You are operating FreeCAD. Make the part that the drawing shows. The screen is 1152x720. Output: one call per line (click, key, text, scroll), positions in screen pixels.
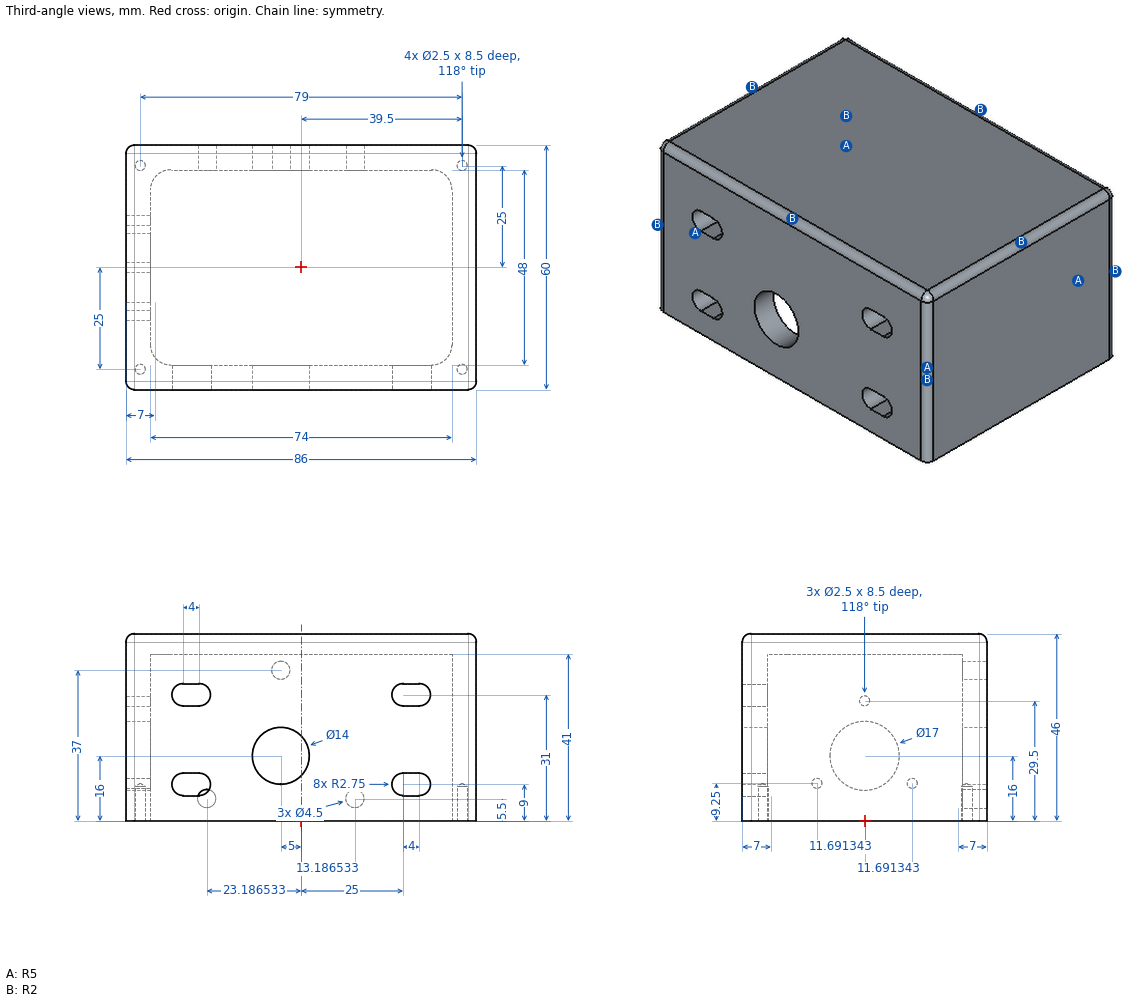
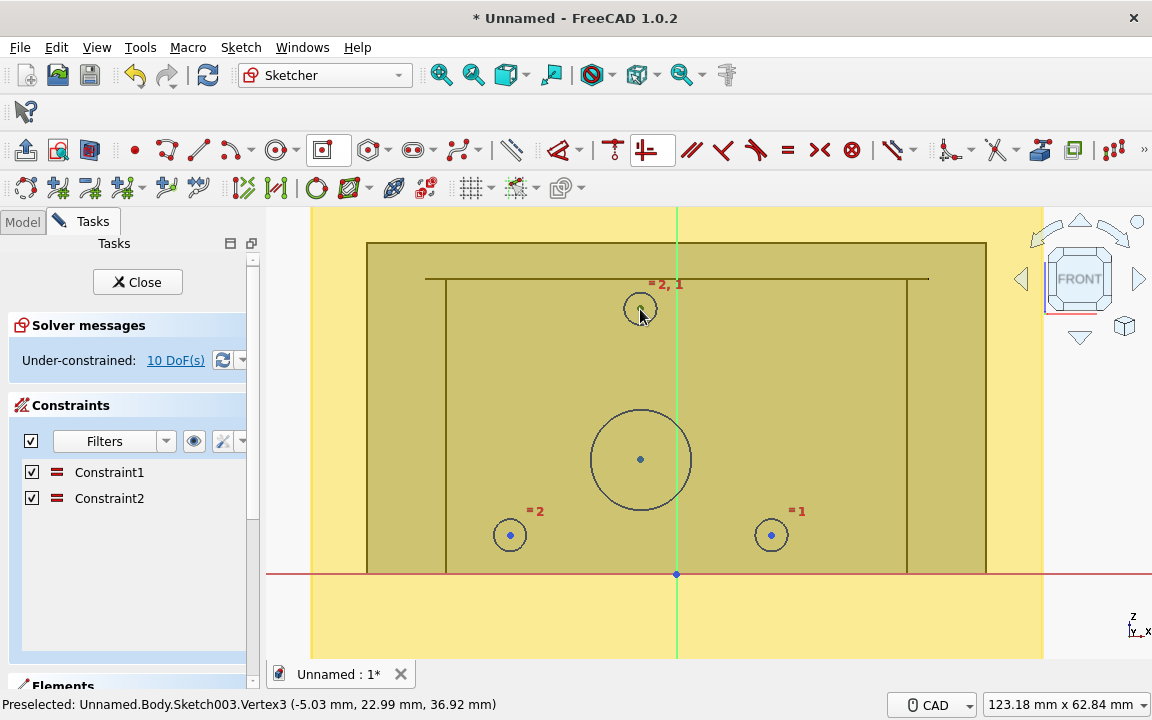
key(v)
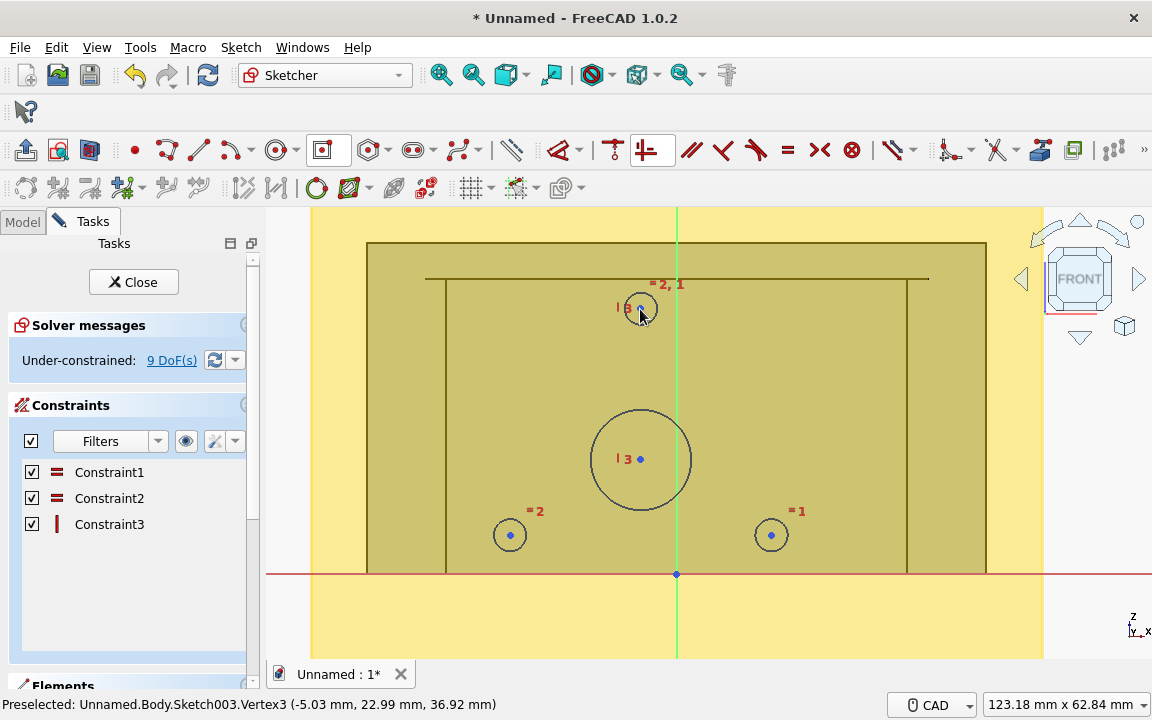
click(772, 535)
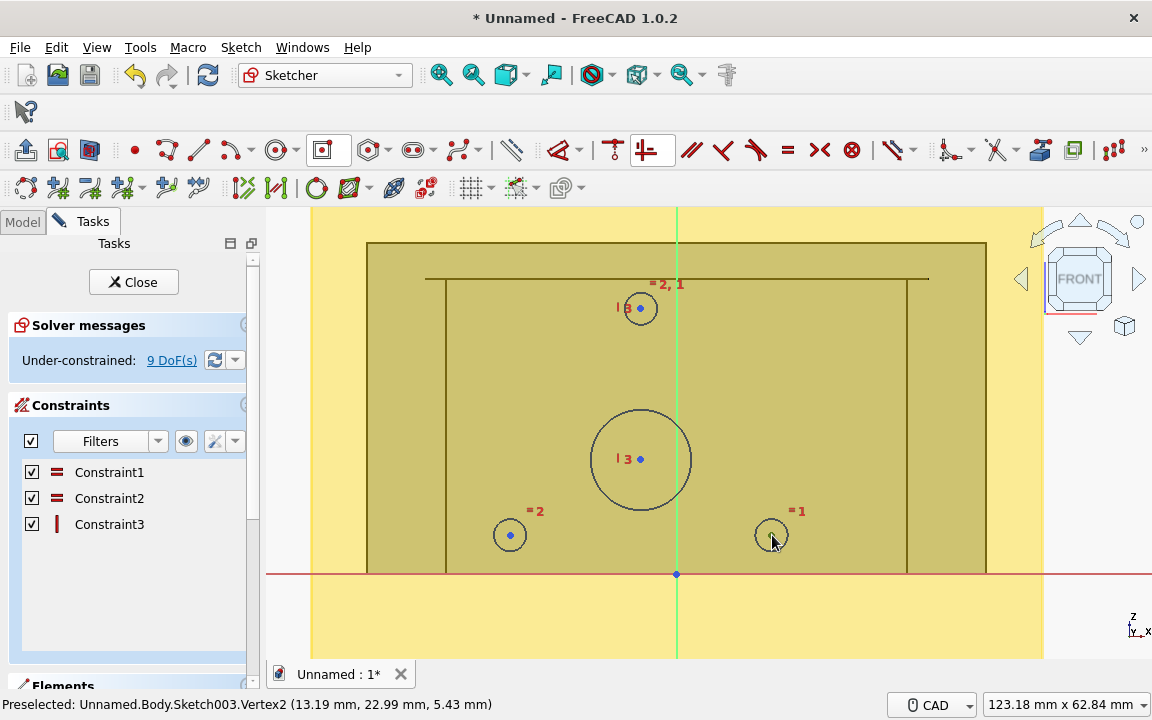
click(510, 535)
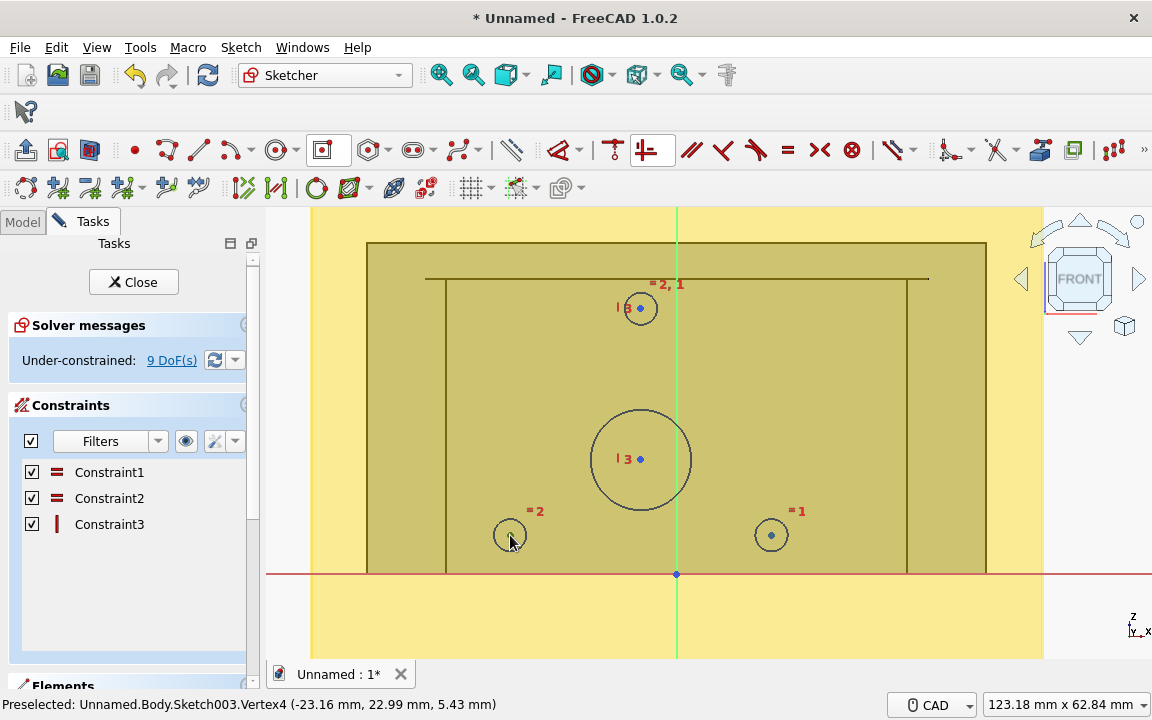
key(h)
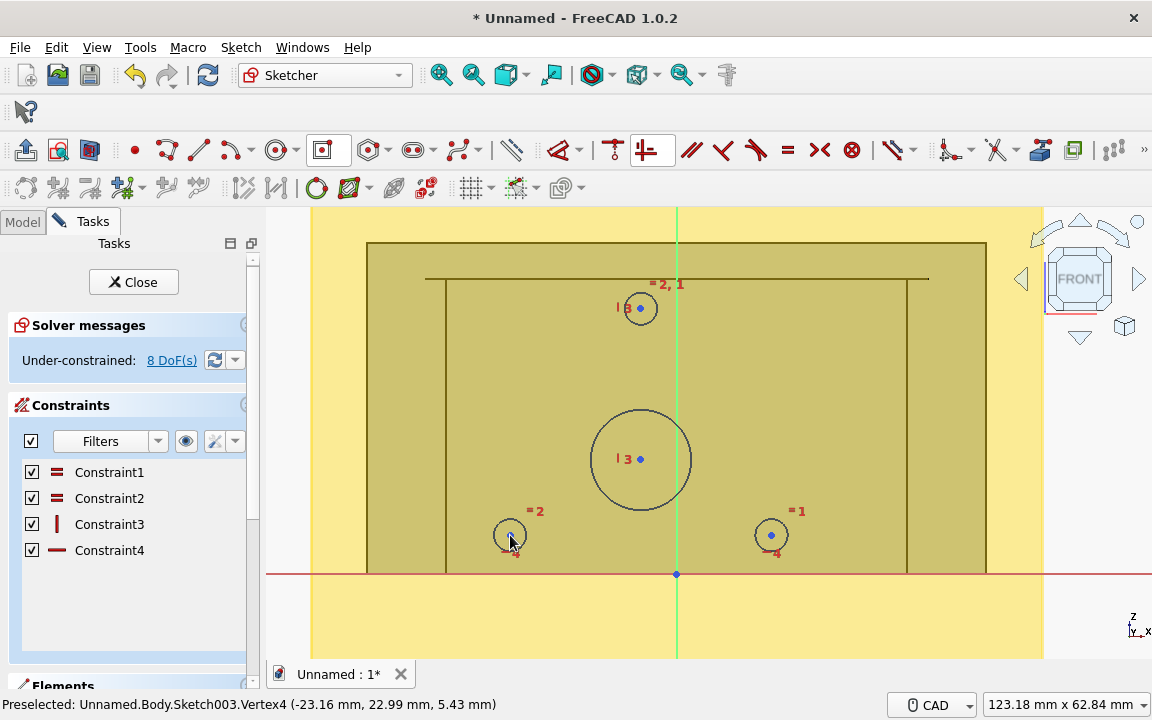
key(d)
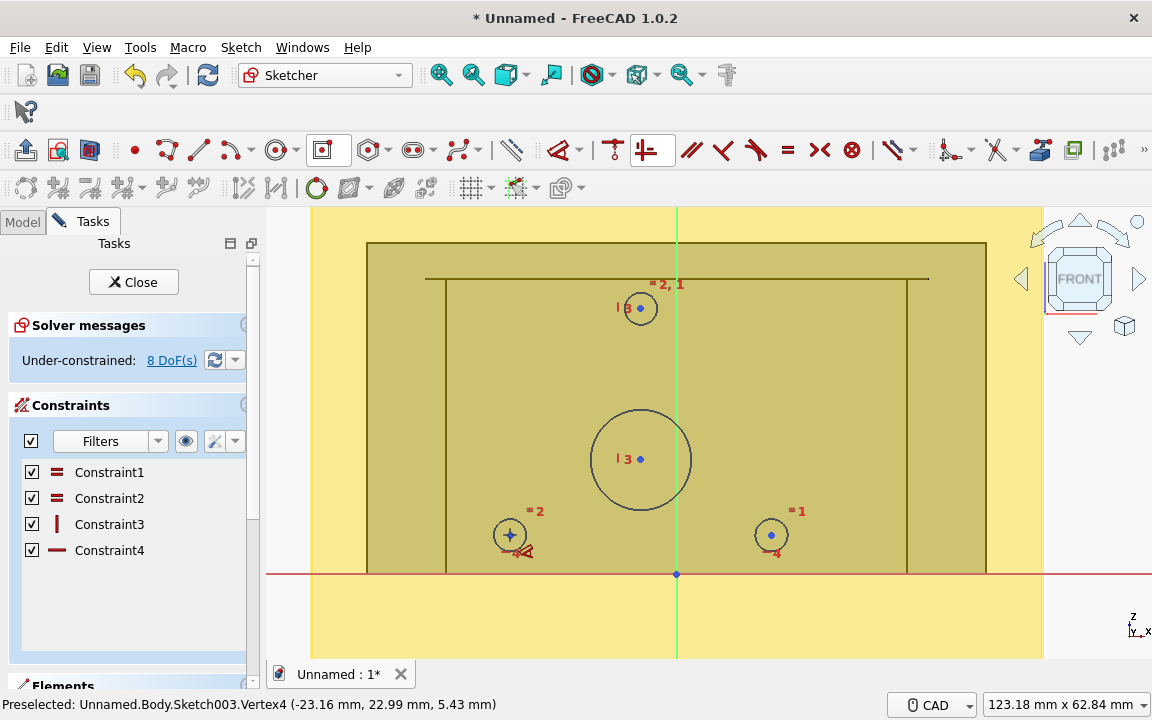
click(676, 424)
click(698, 401)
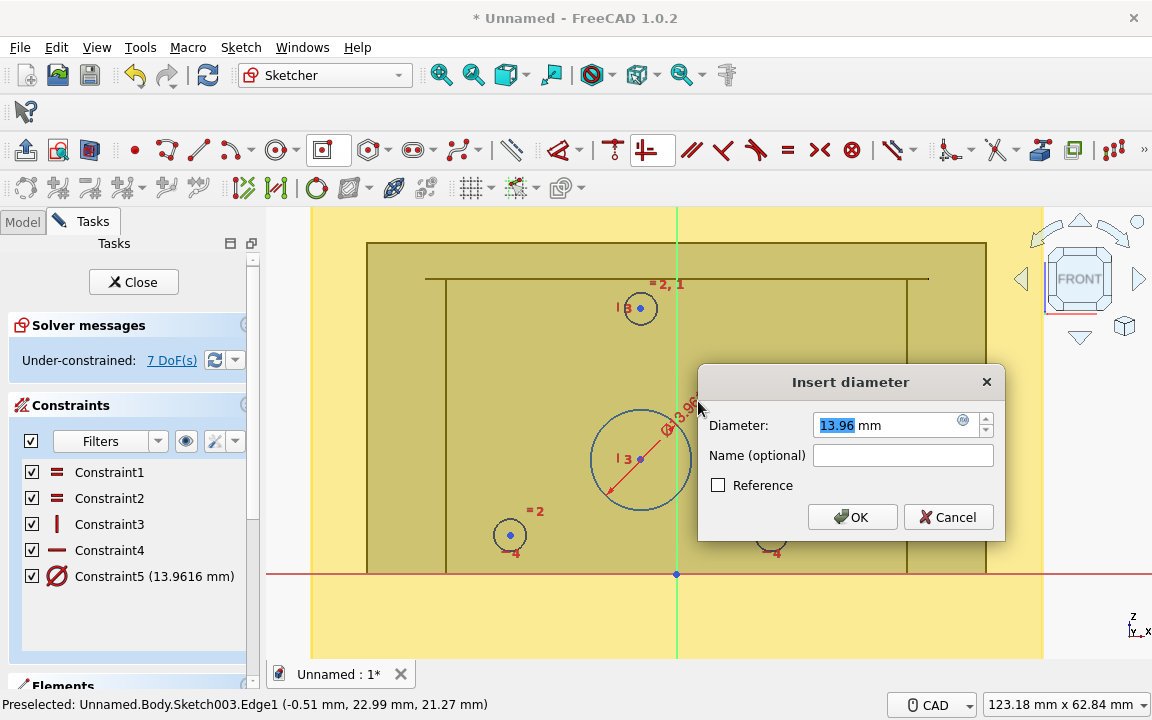
text(14)
key(Return)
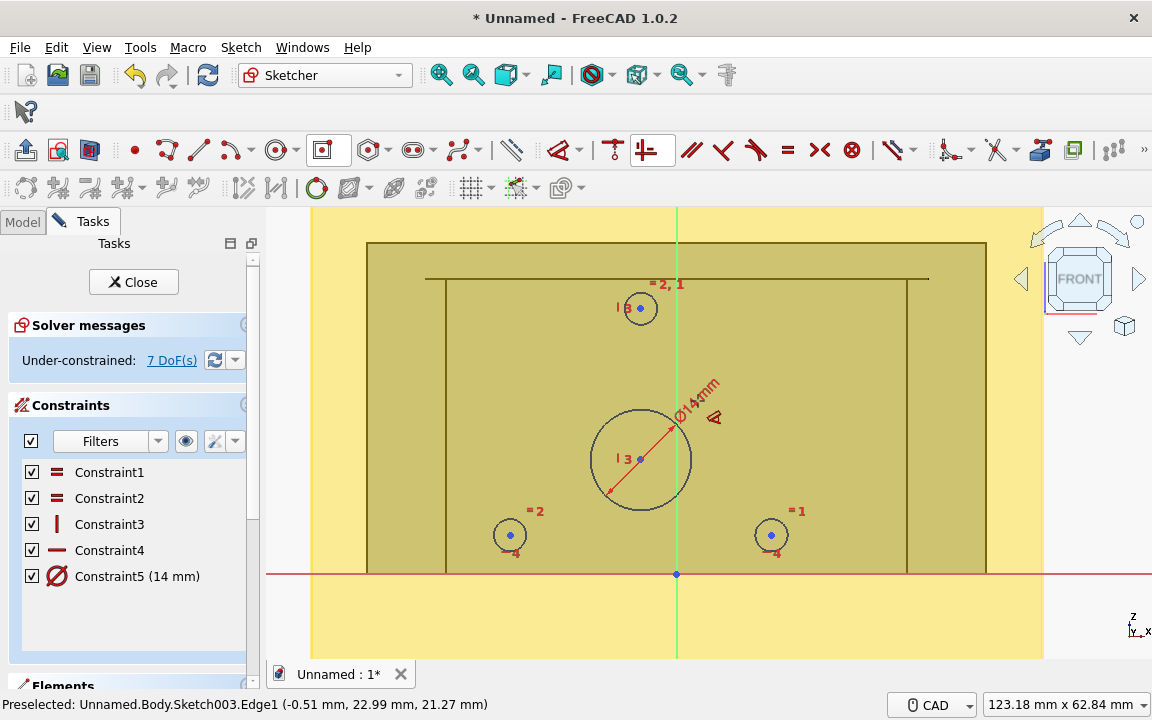
scroll(783, 524, up, 2)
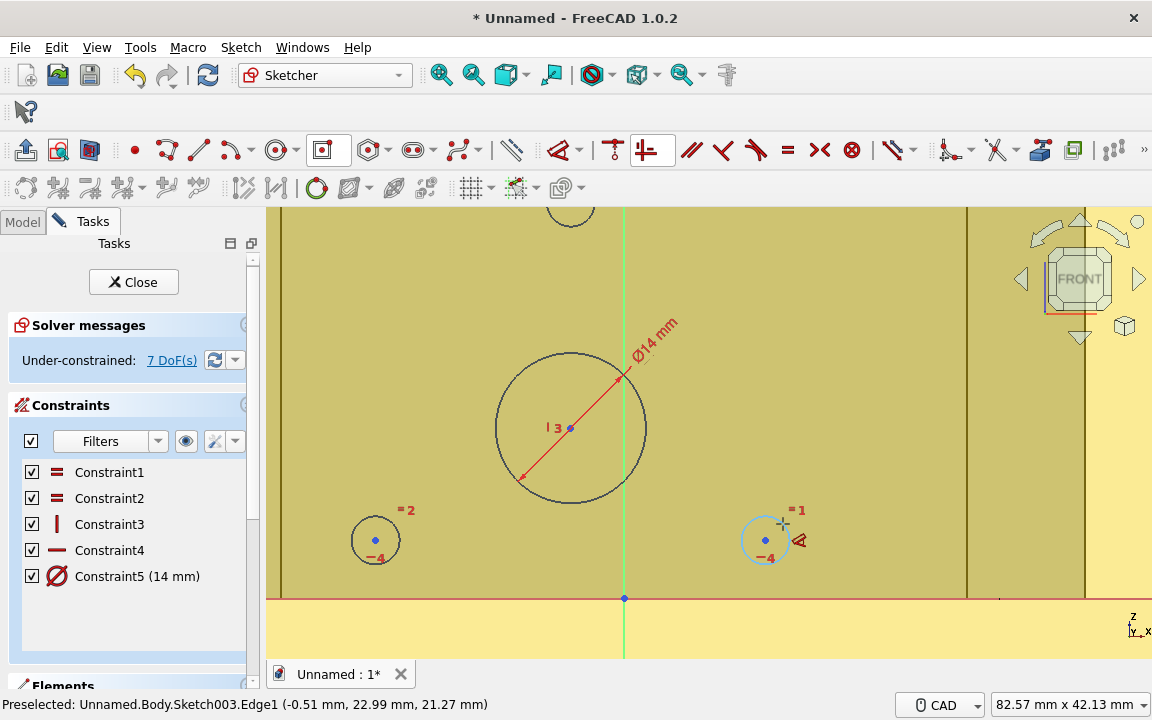
click(783, 523)
click(806, 500)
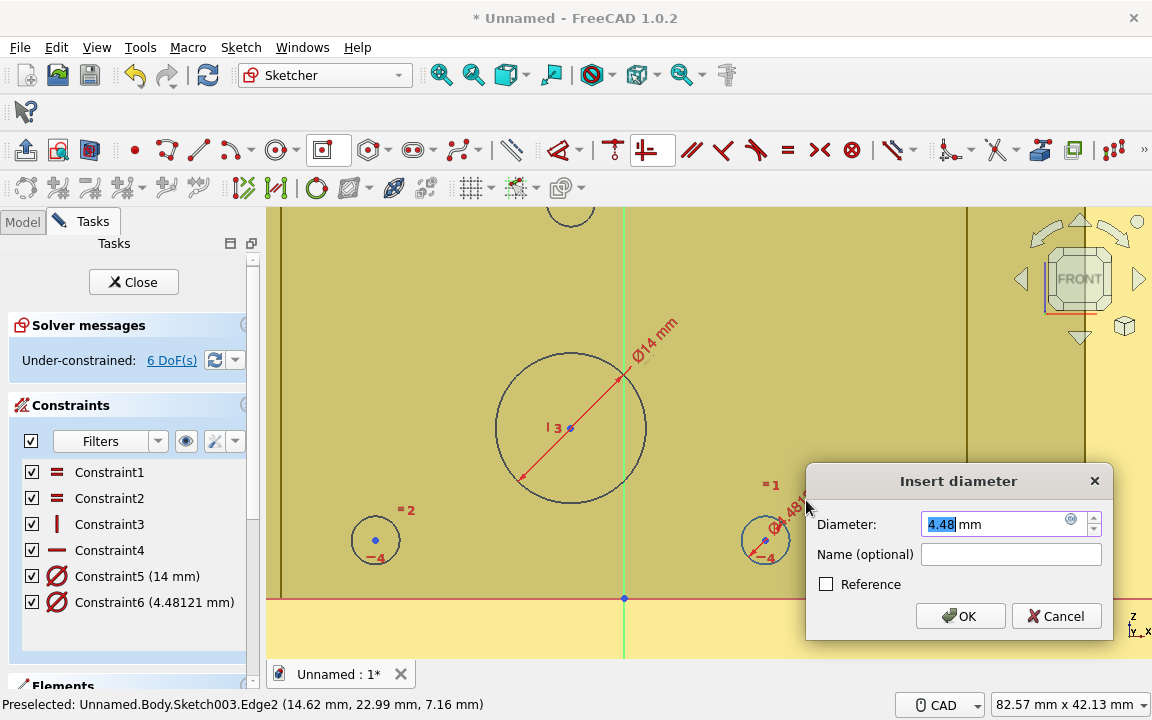
text(4.5)
key(Return)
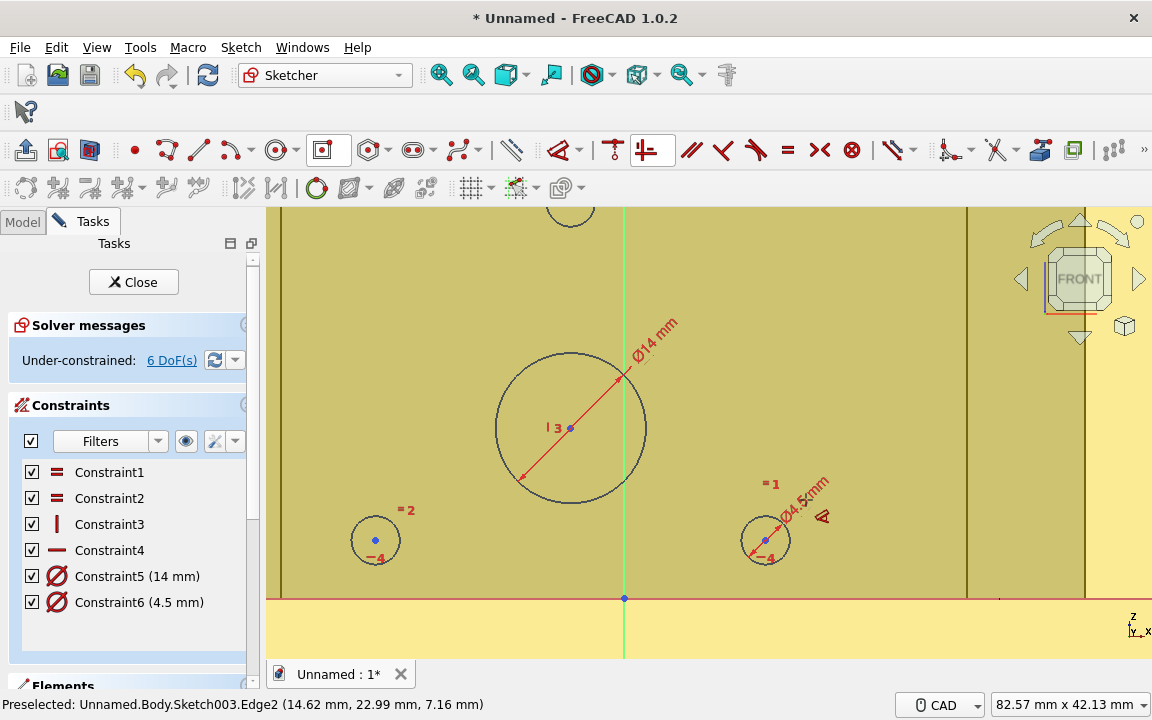
click(571, 428)
click(597, 394)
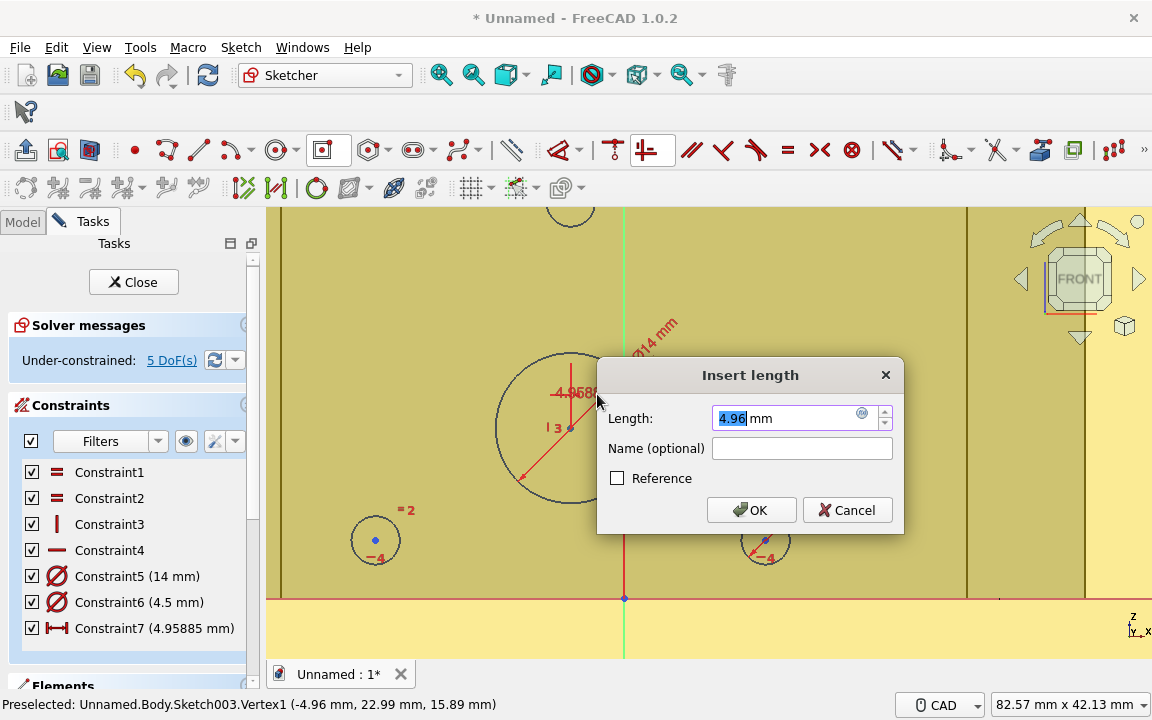
text(5)
key(Return)